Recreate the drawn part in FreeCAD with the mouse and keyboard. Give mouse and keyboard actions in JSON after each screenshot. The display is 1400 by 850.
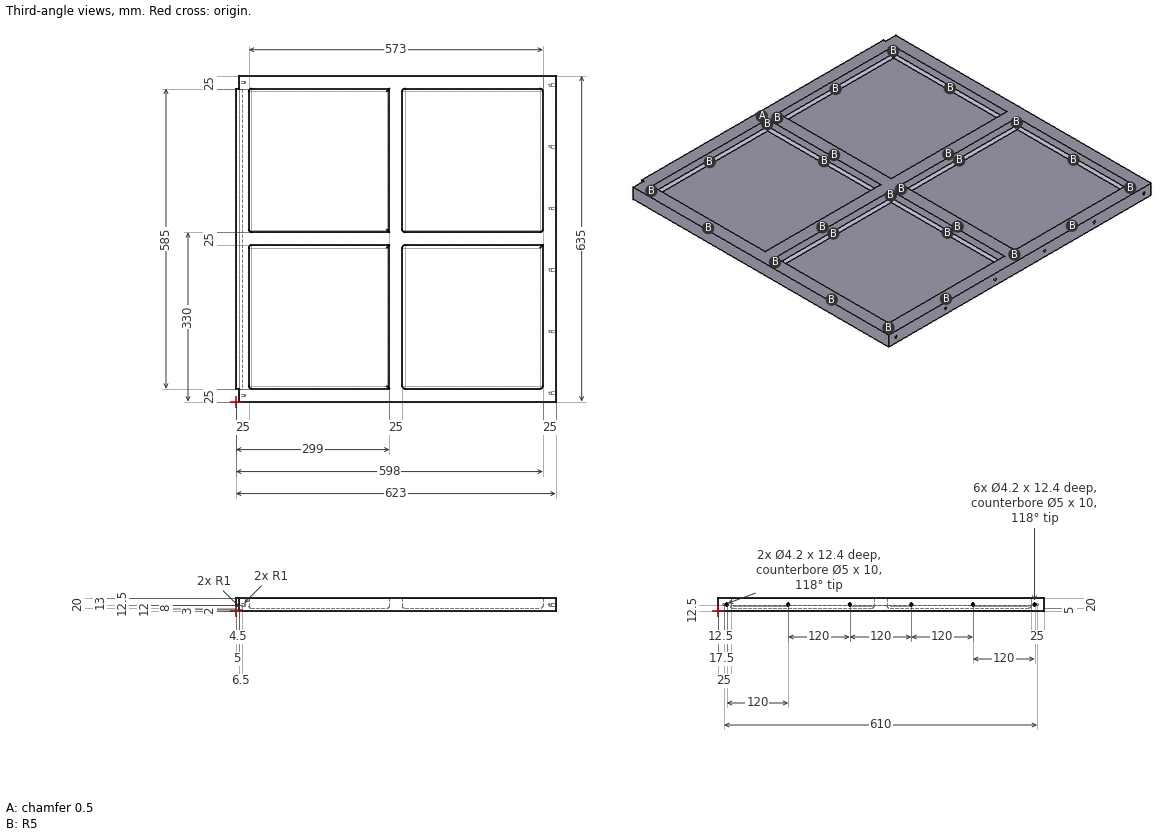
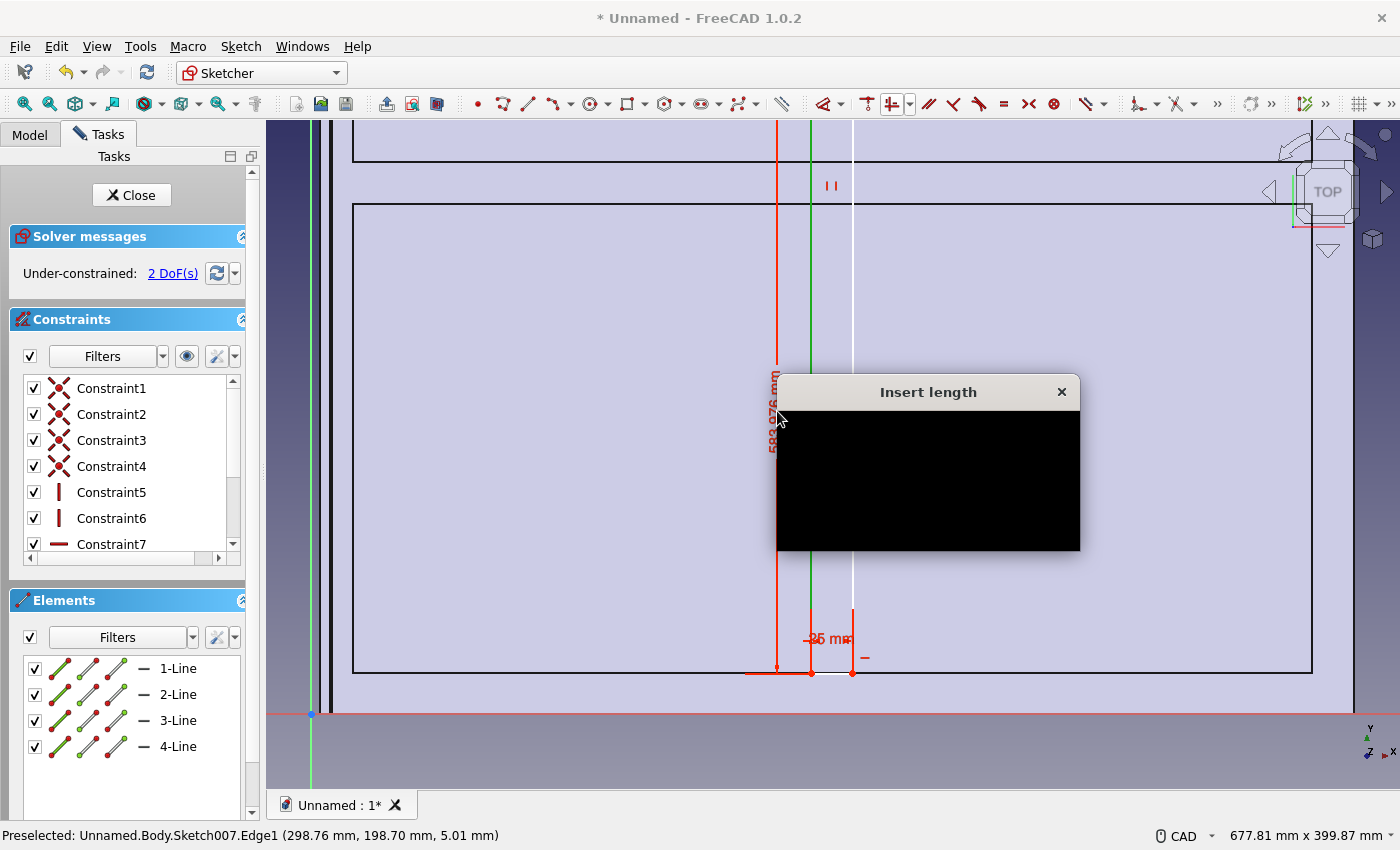
{"action": "type", "text": "585"}
{"action": "key", "text": "Return"}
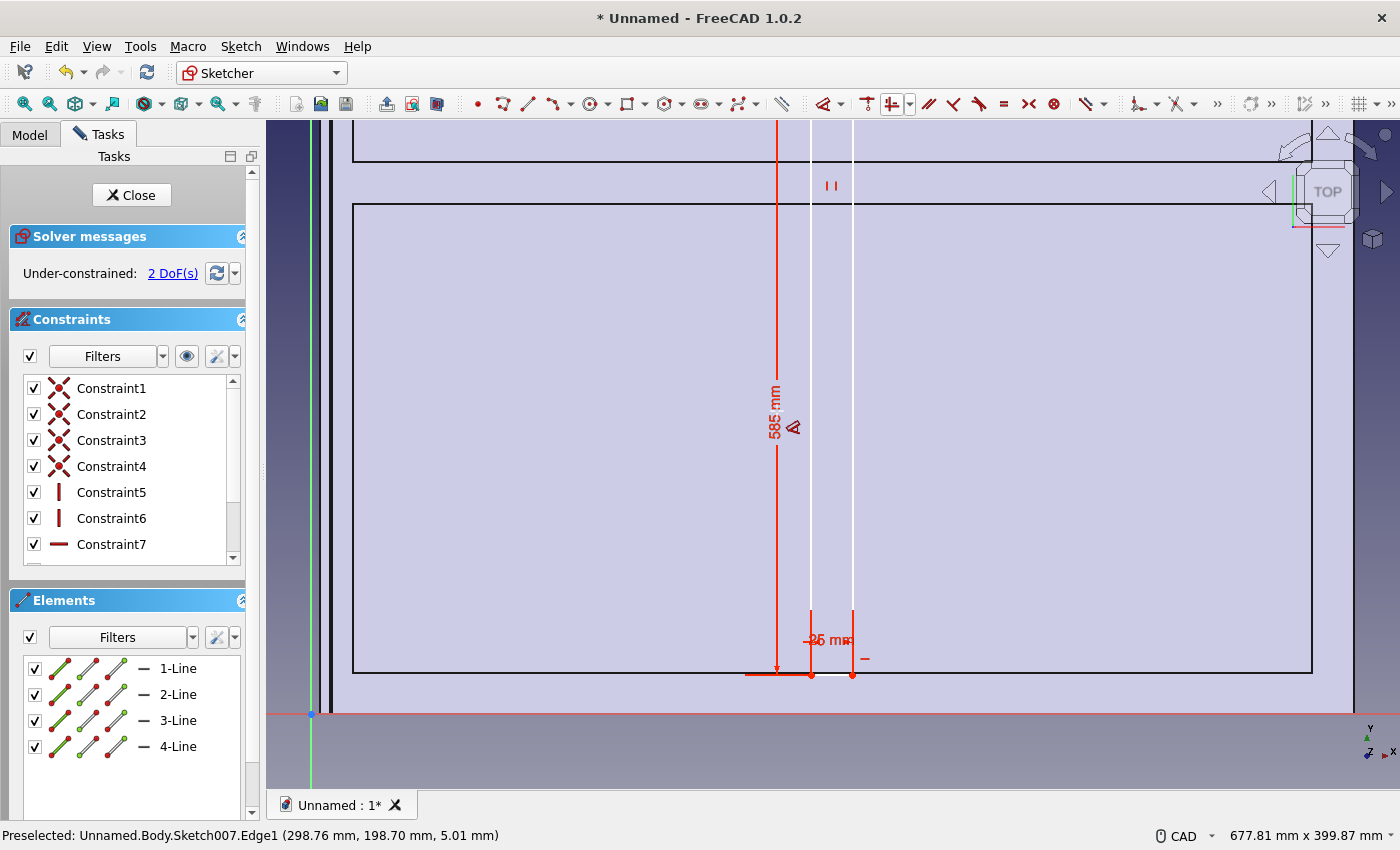
{"action": "left_click", "coordinate": [811, 675]}
{"action": "left_click", "coordinate": [845, 695]}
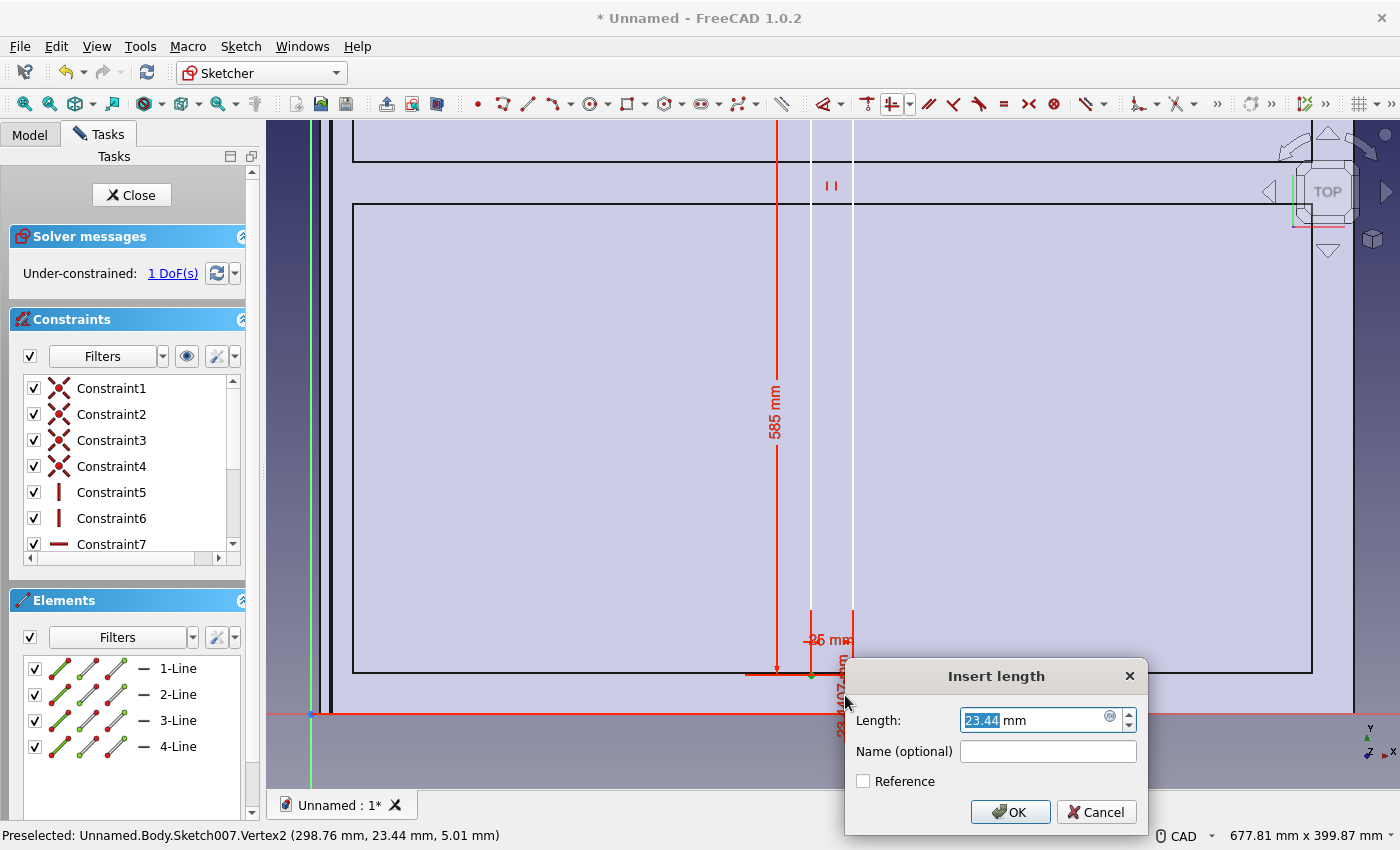
{"action": "type", "text": "25"}
{"action": "key", "text": "Return"}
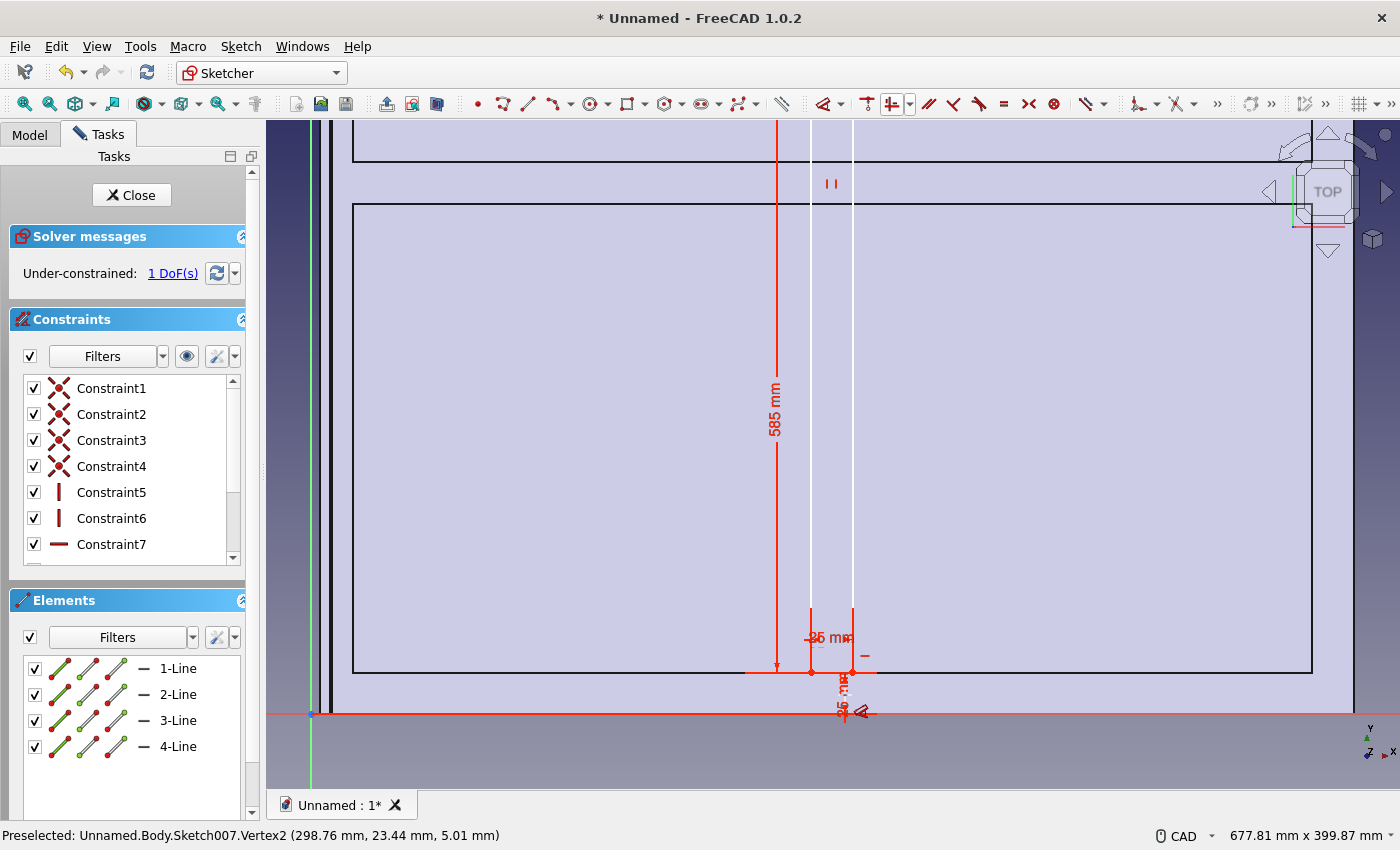
{"action": "scroll", "coordinate": [913, 659], "scroll_direction": "down", "scroll_amount": 4}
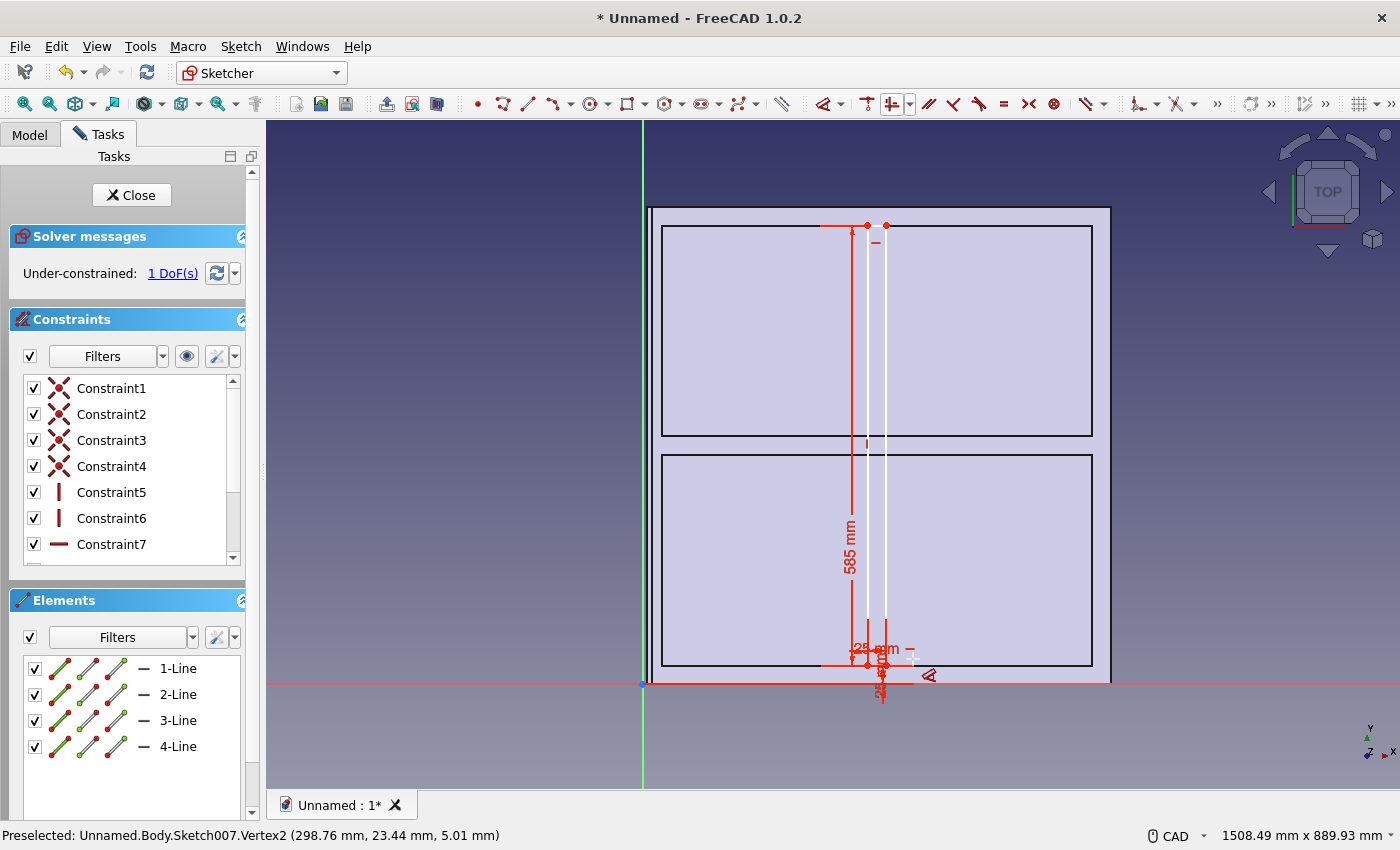
{"action": "left_click", "coordinate": [868, 226]}
{"action": "left_click", "coordinate": [755, 718]}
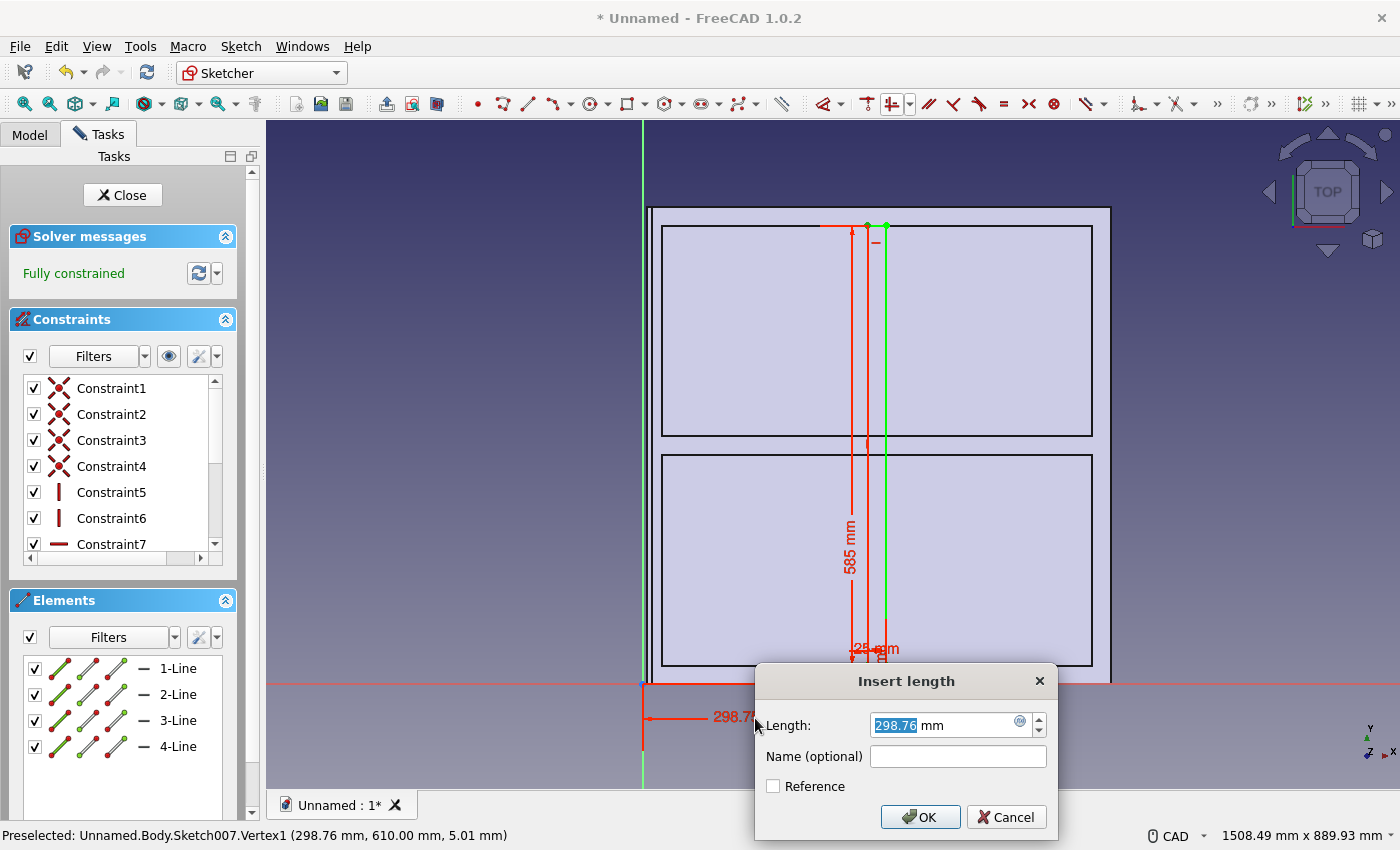
{"action": "type", "text": "299"}
{"action": "key", "text": "Return"}
{"action": "key", "text": "Escape"}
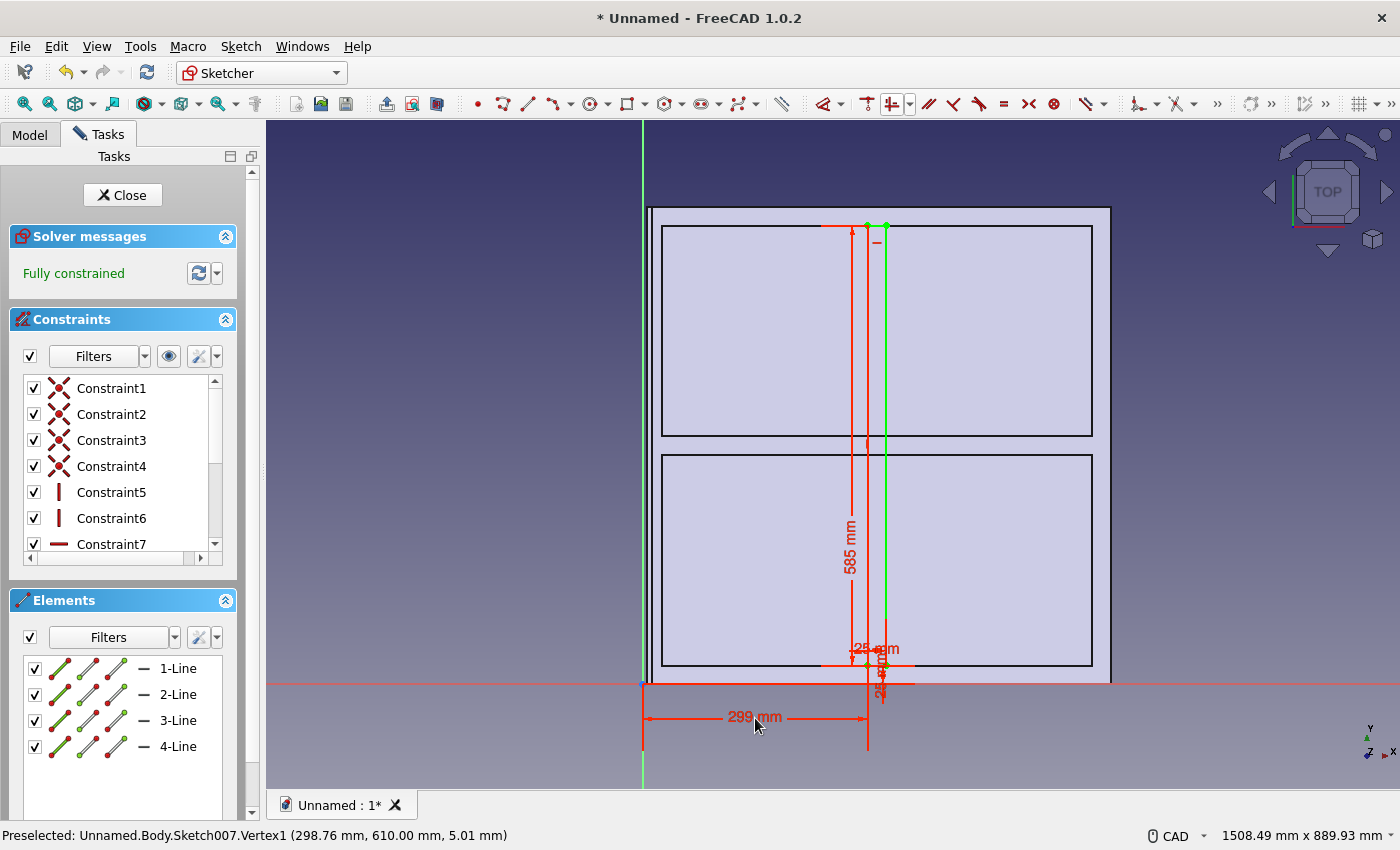
{"action": "left_click", "coordinate": [123, 195]}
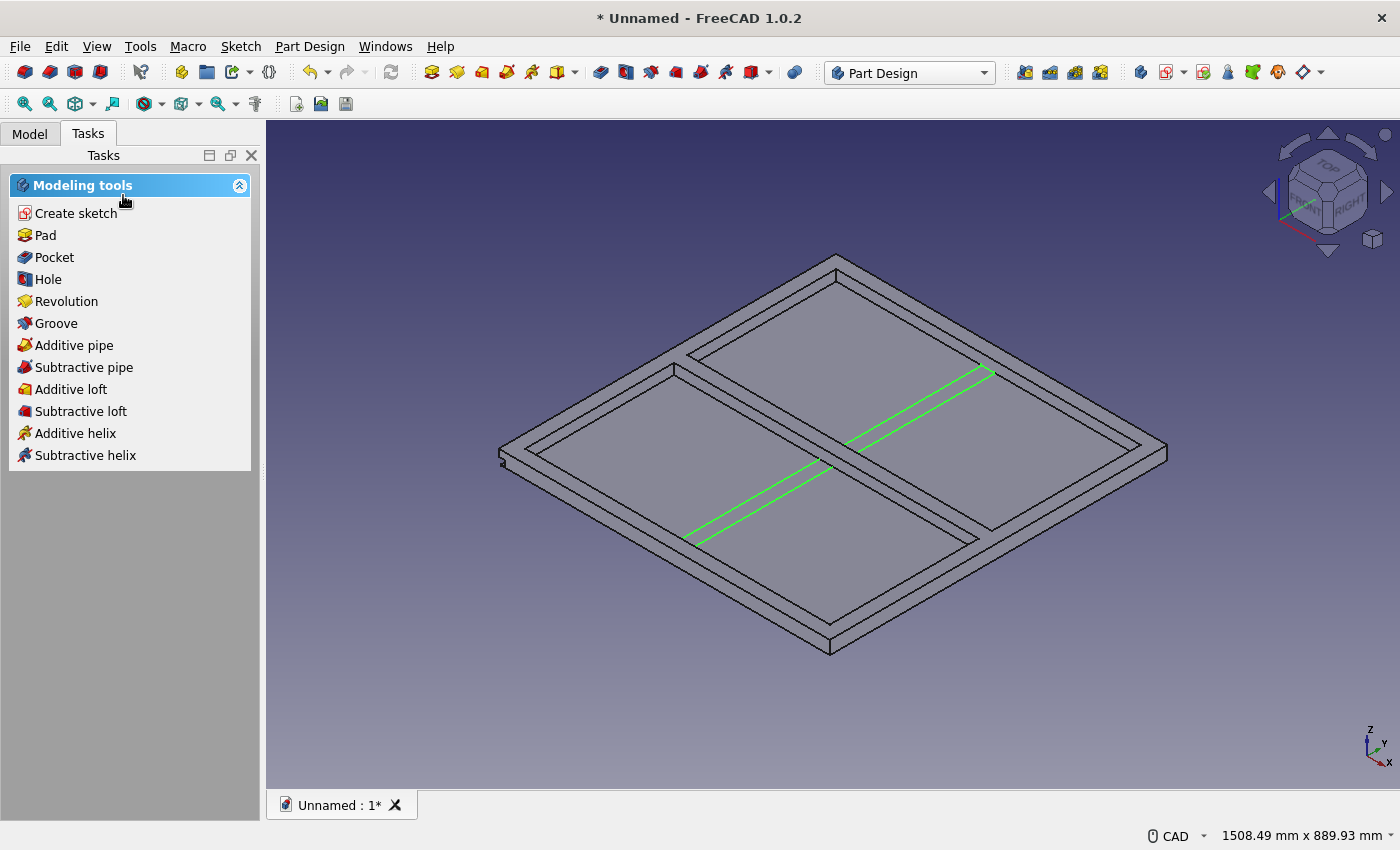
{"action": "left_click", "coordinate": [432, 72]}